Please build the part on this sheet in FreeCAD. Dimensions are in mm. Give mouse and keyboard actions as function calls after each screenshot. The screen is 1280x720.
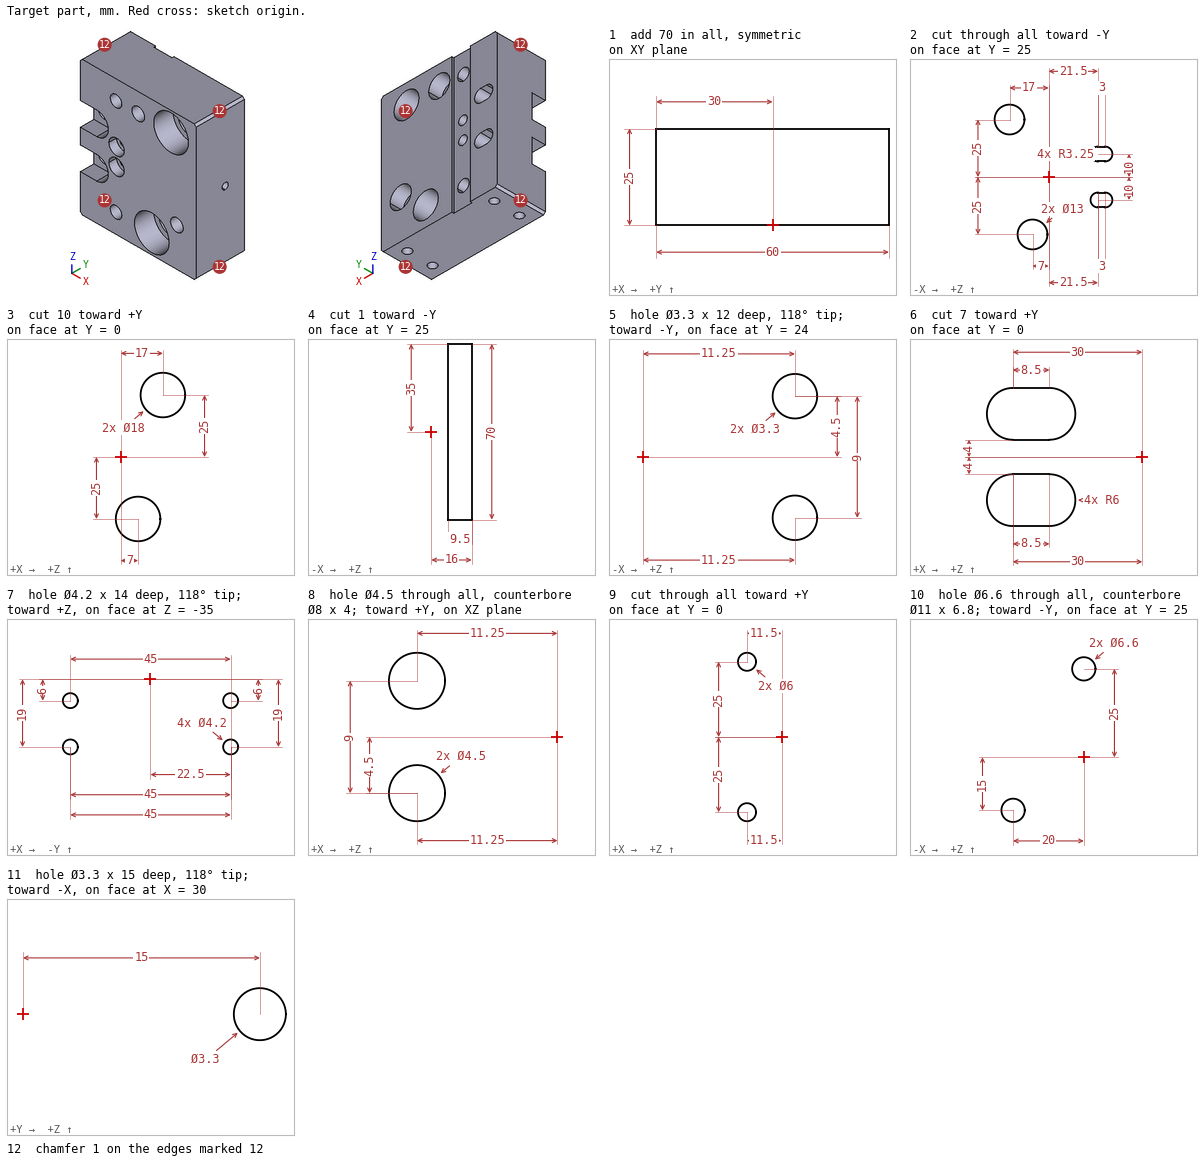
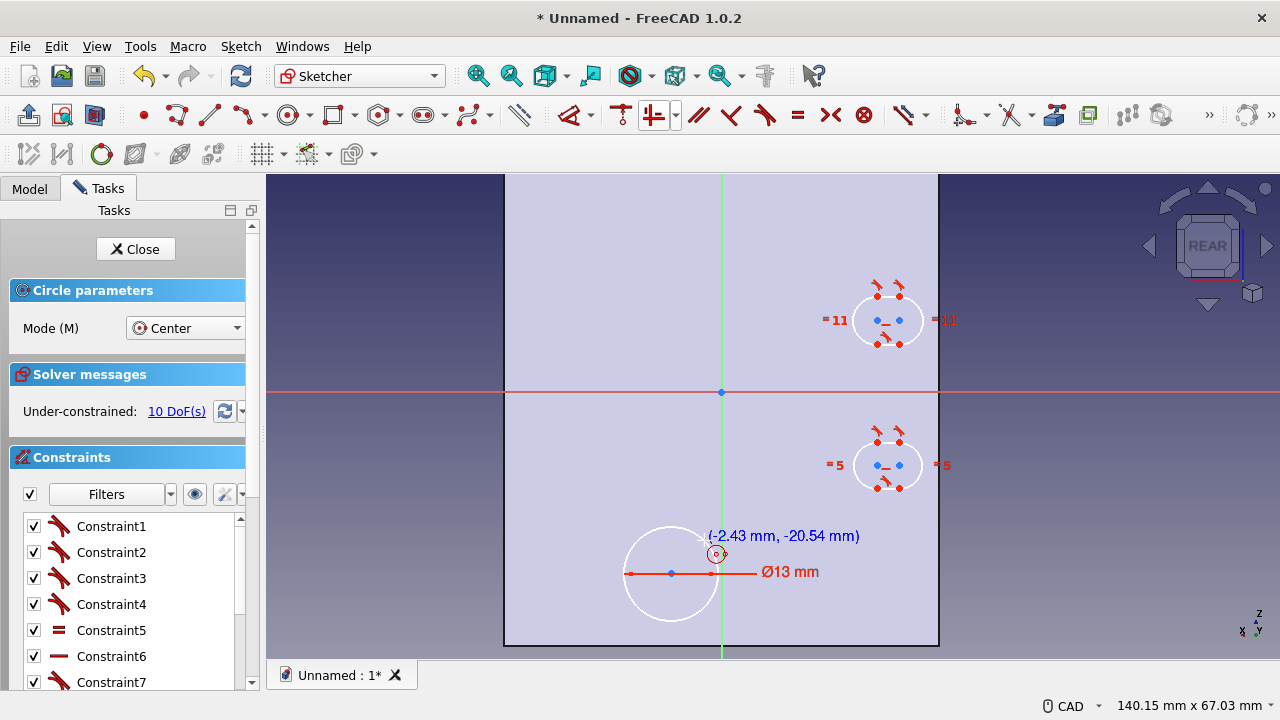
click(599, 211)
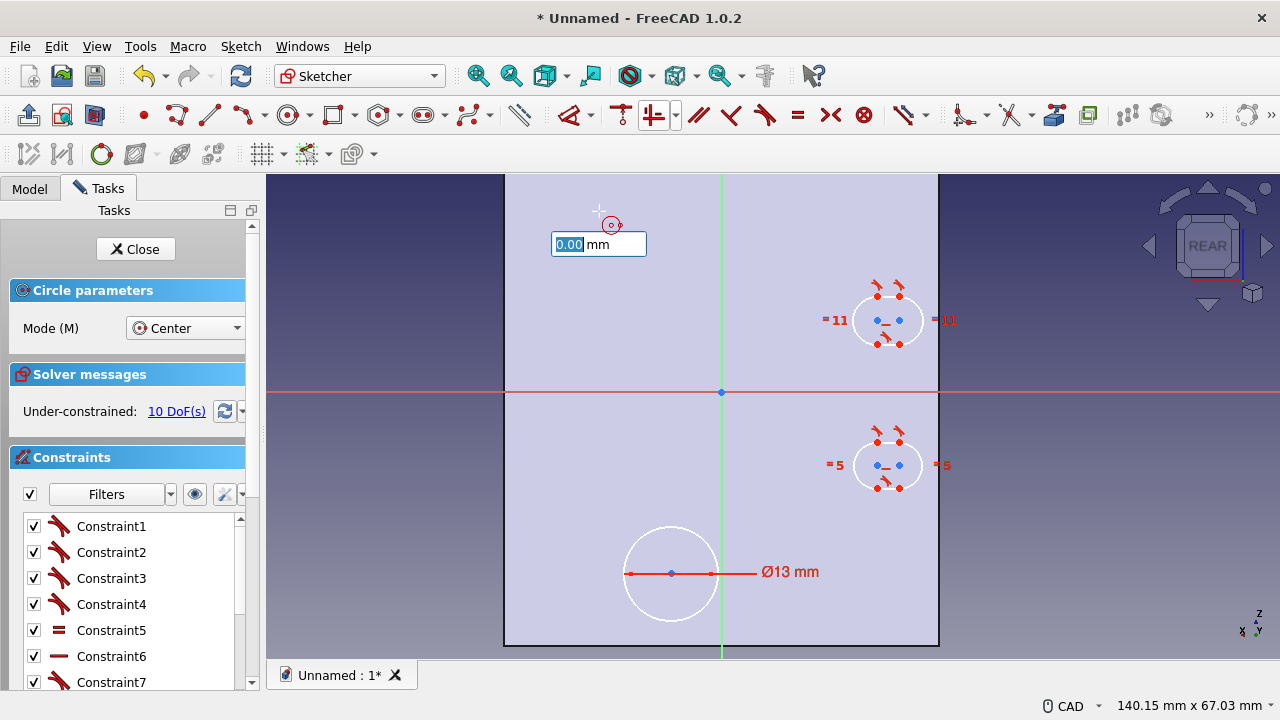
scroll(639, 466, down, 2)
move(634, 273)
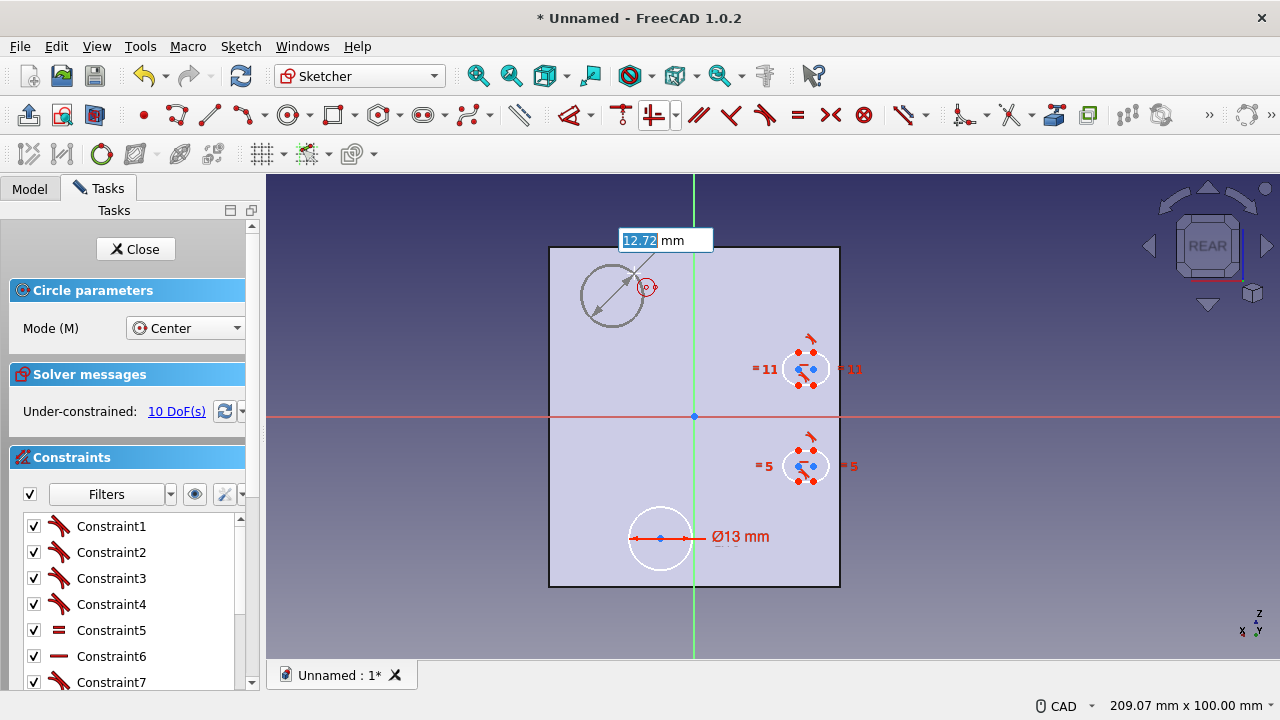
text(13)
key(Return)
key(Escape)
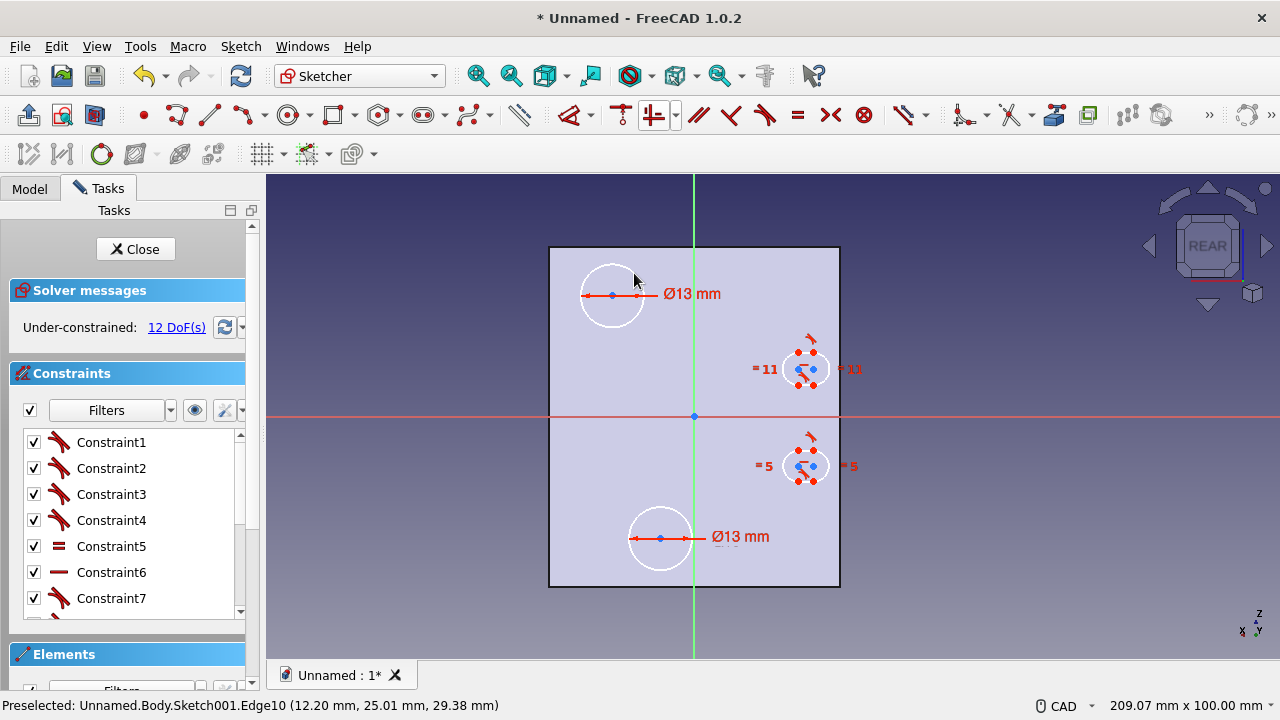
click(786, 457)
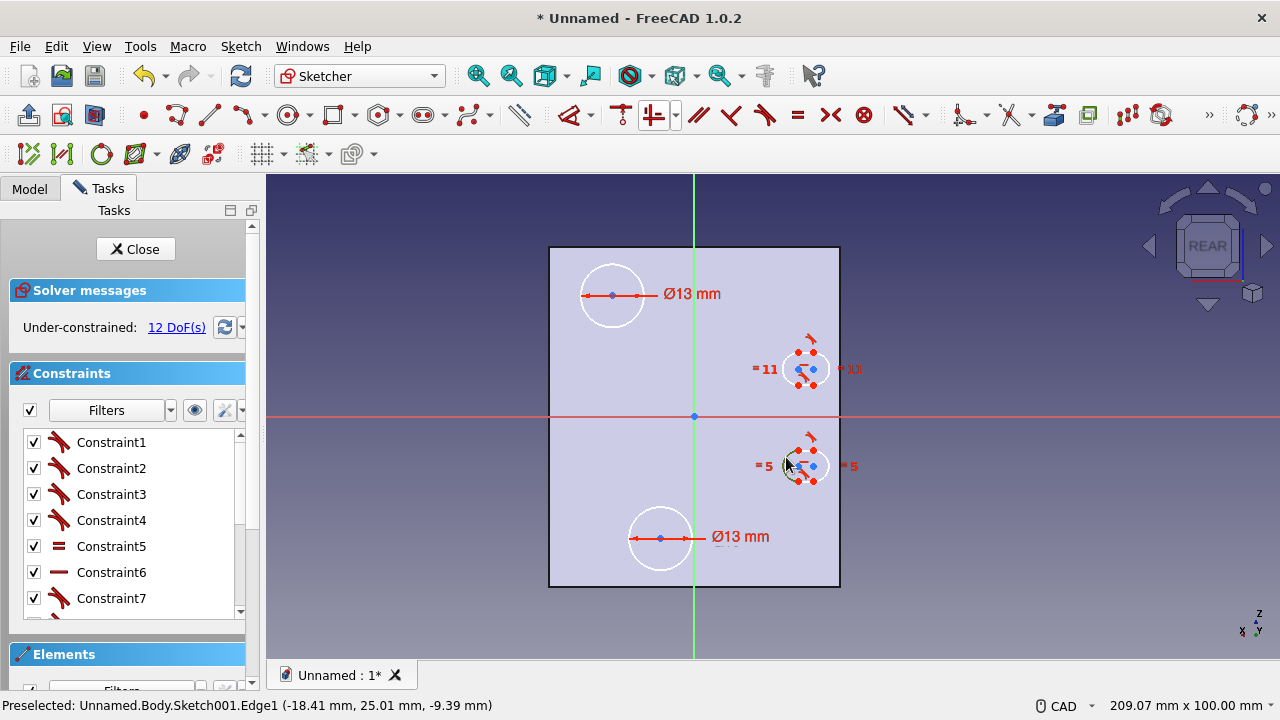
click(786, 360)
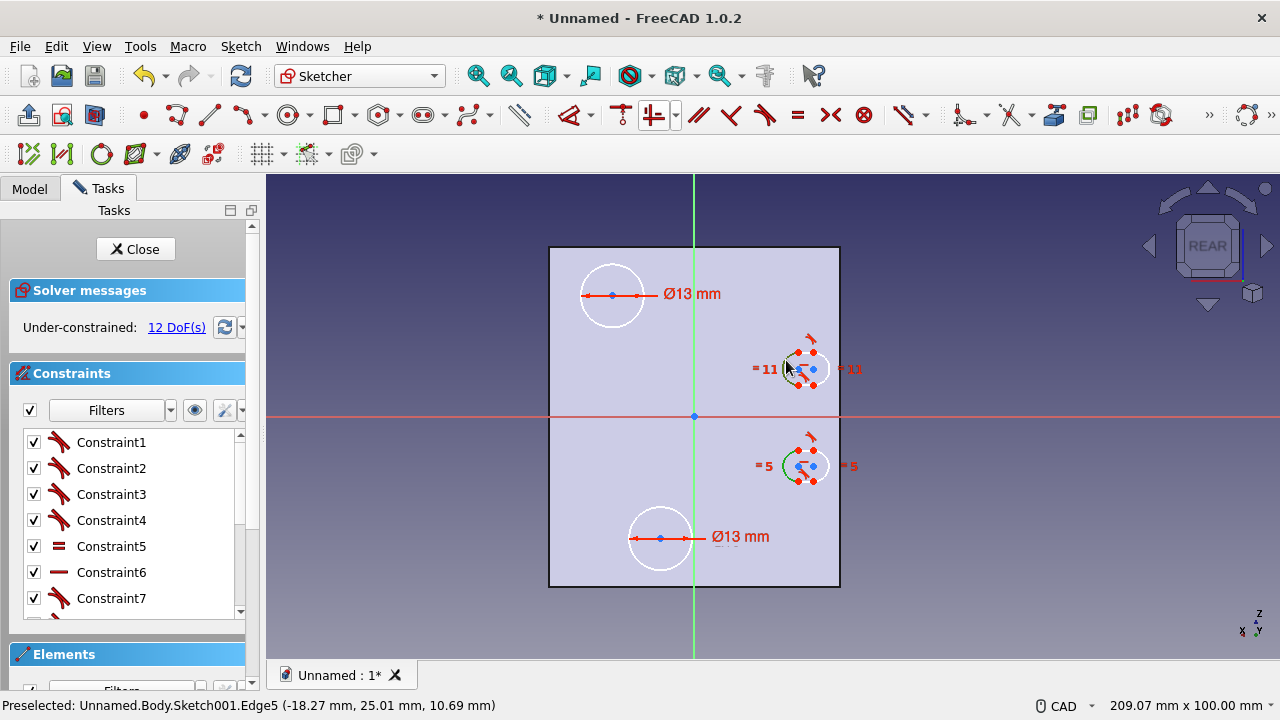
key(e)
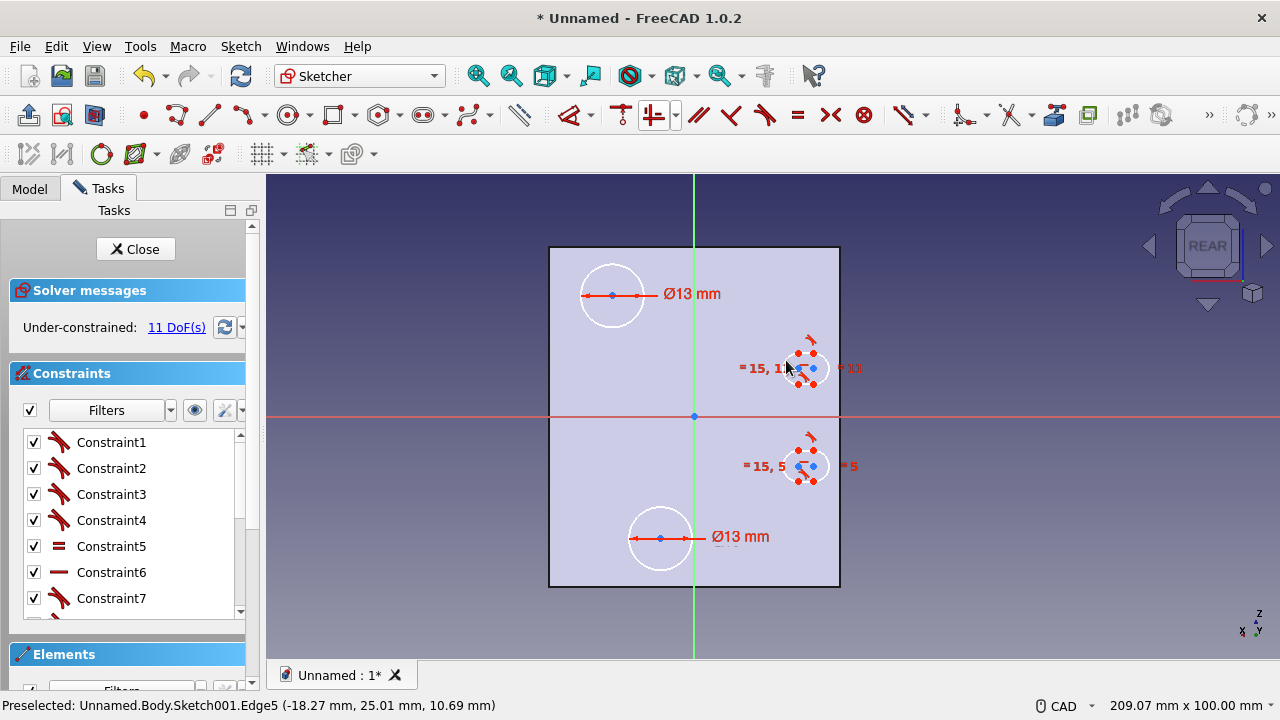
key(d)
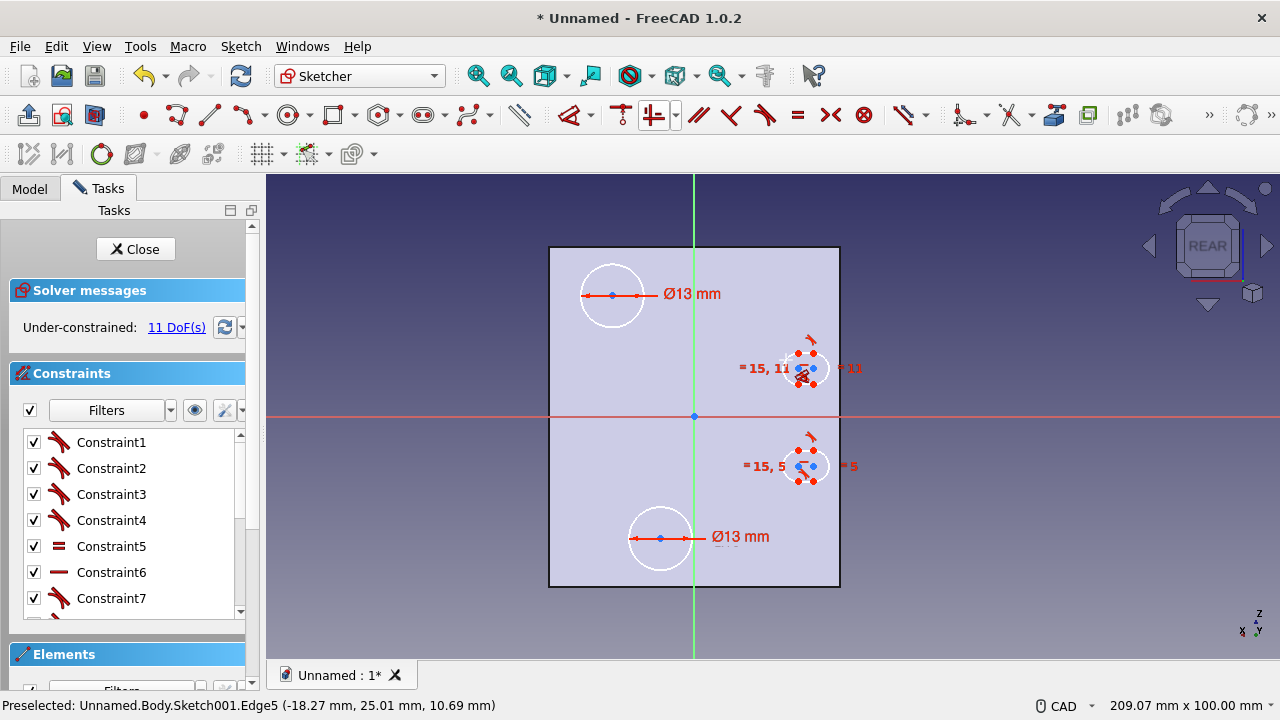
scroll(786, 457, up, 5)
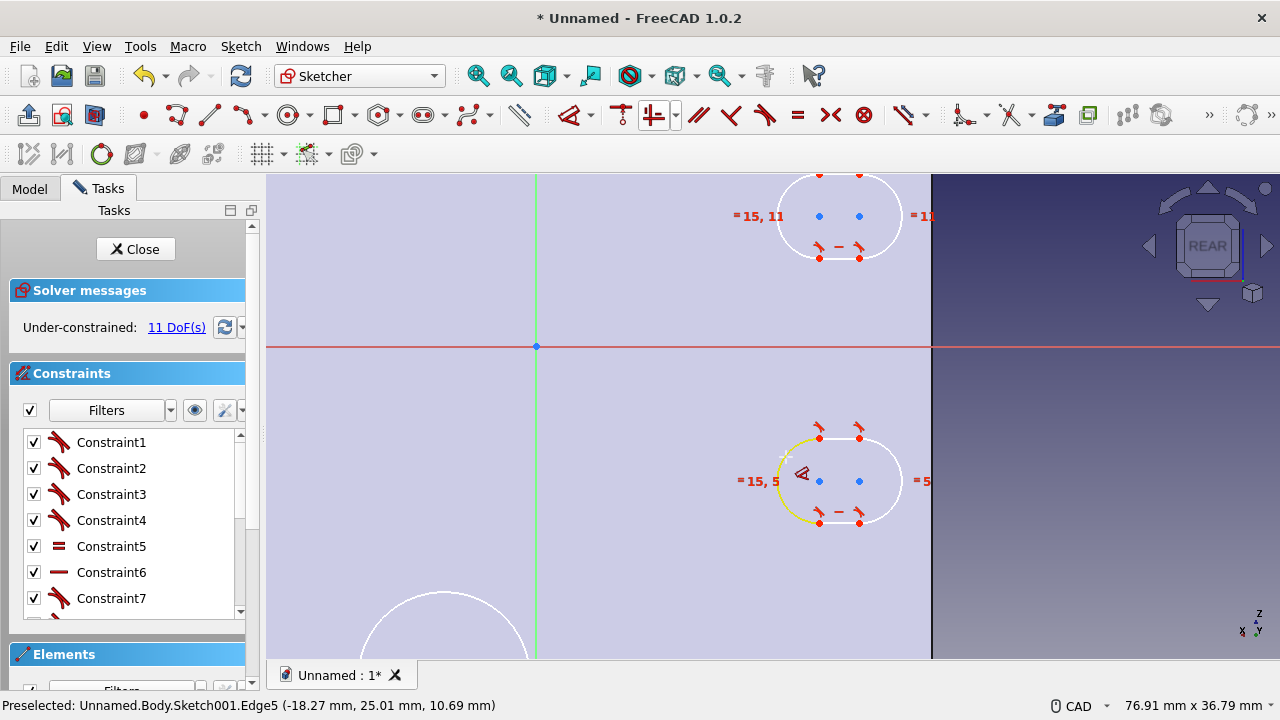
click(785, 456)
click(759, 437)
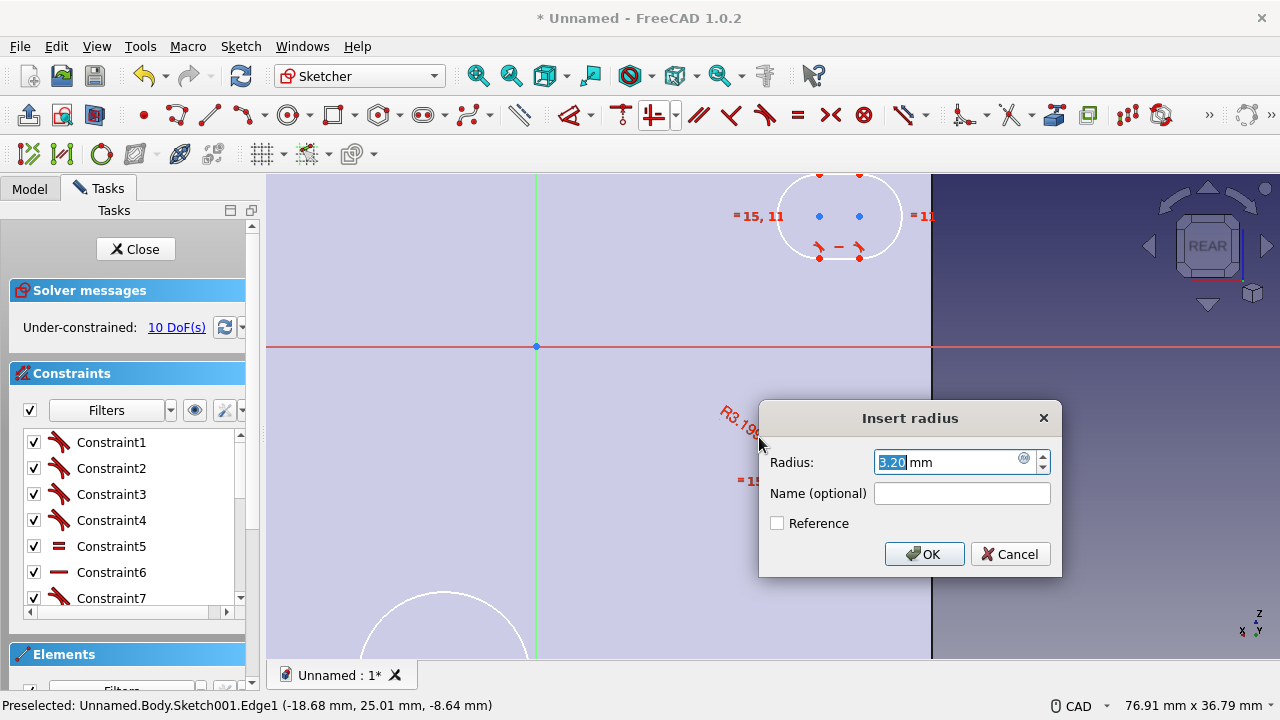
text(3.25)
key(Return)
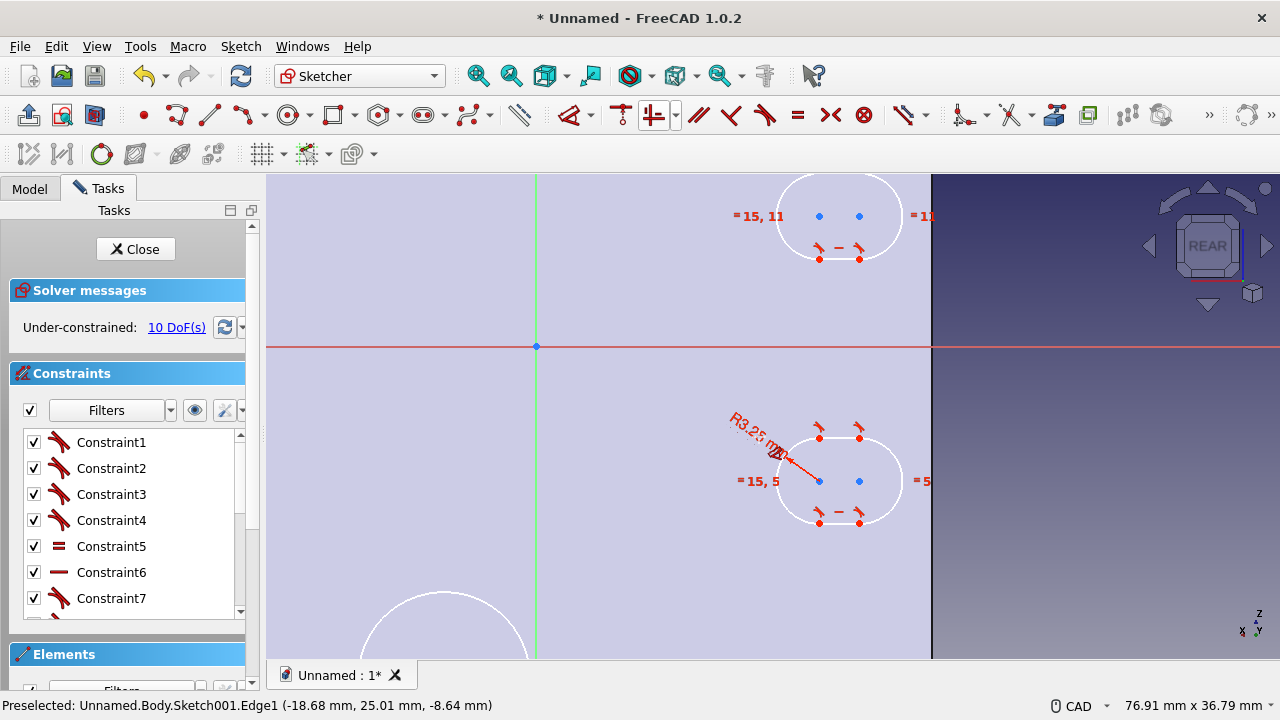
click(832, 438)
click(840, 472)